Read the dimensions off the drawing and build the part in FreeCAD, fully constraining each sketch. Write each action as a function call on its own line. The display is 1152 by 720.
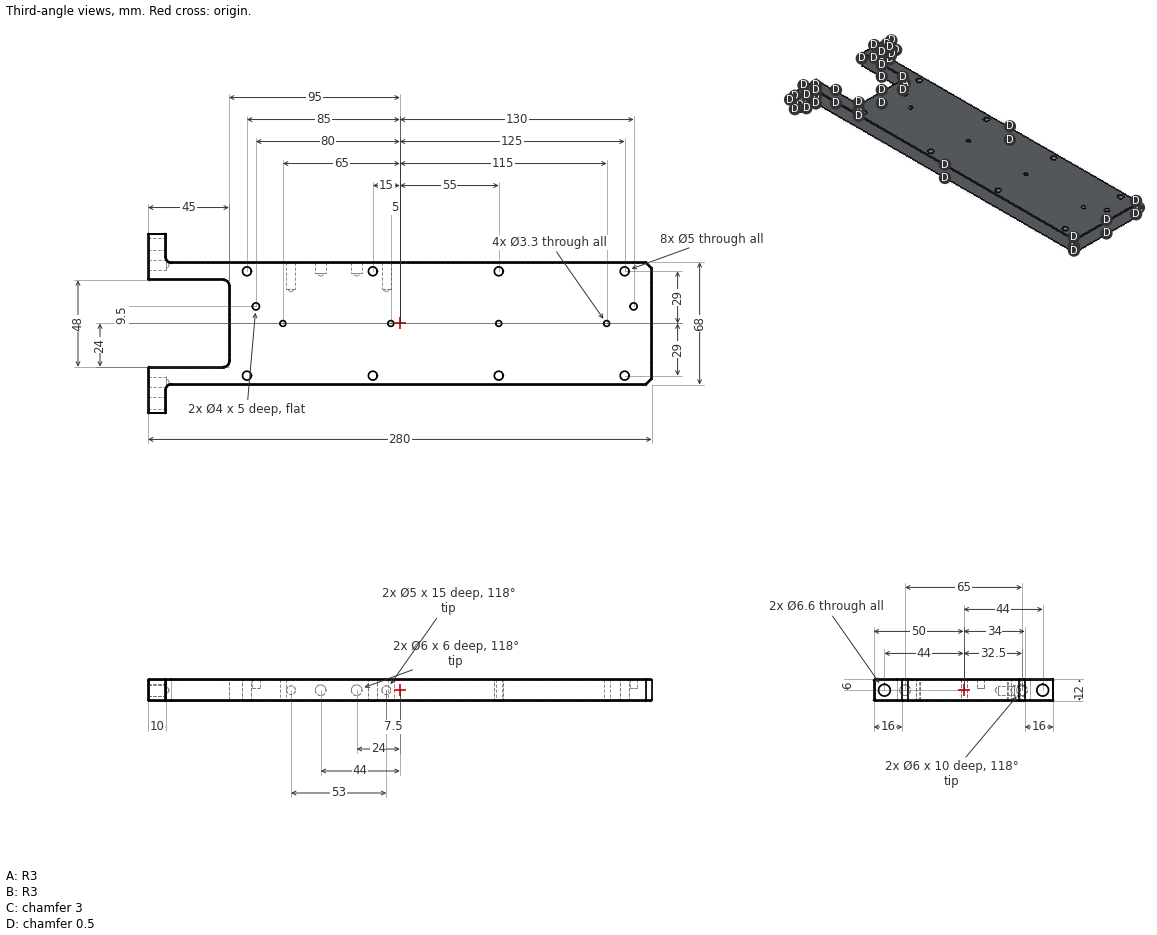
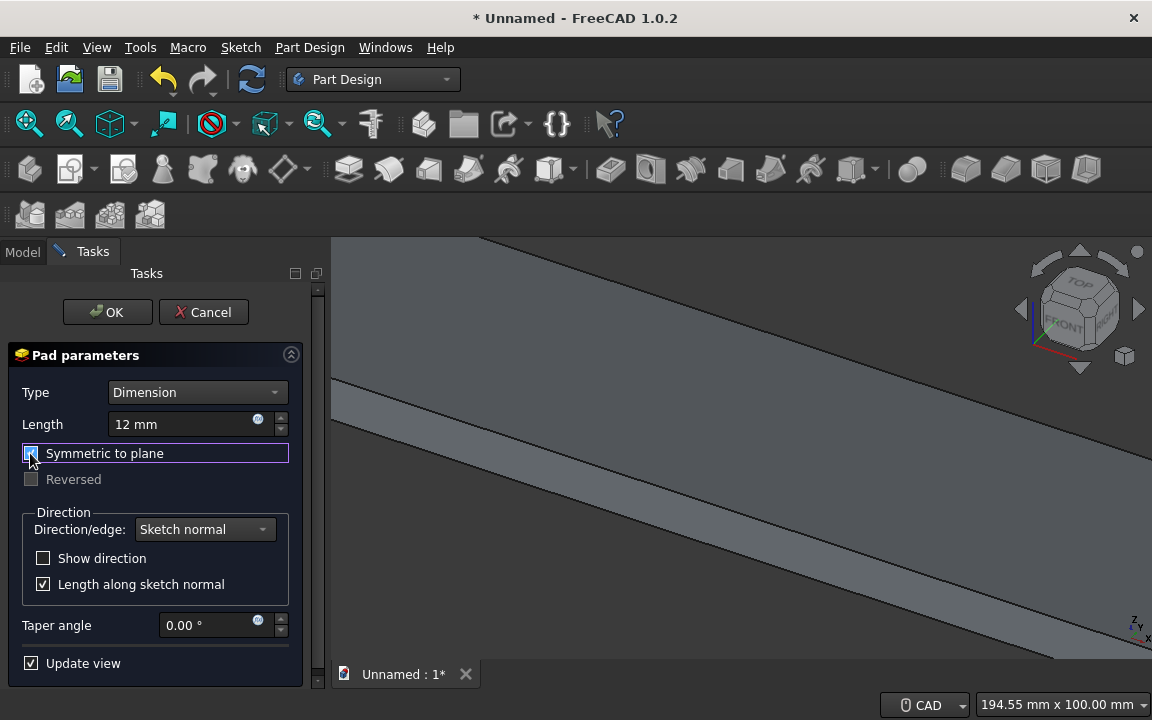
click(108, 312)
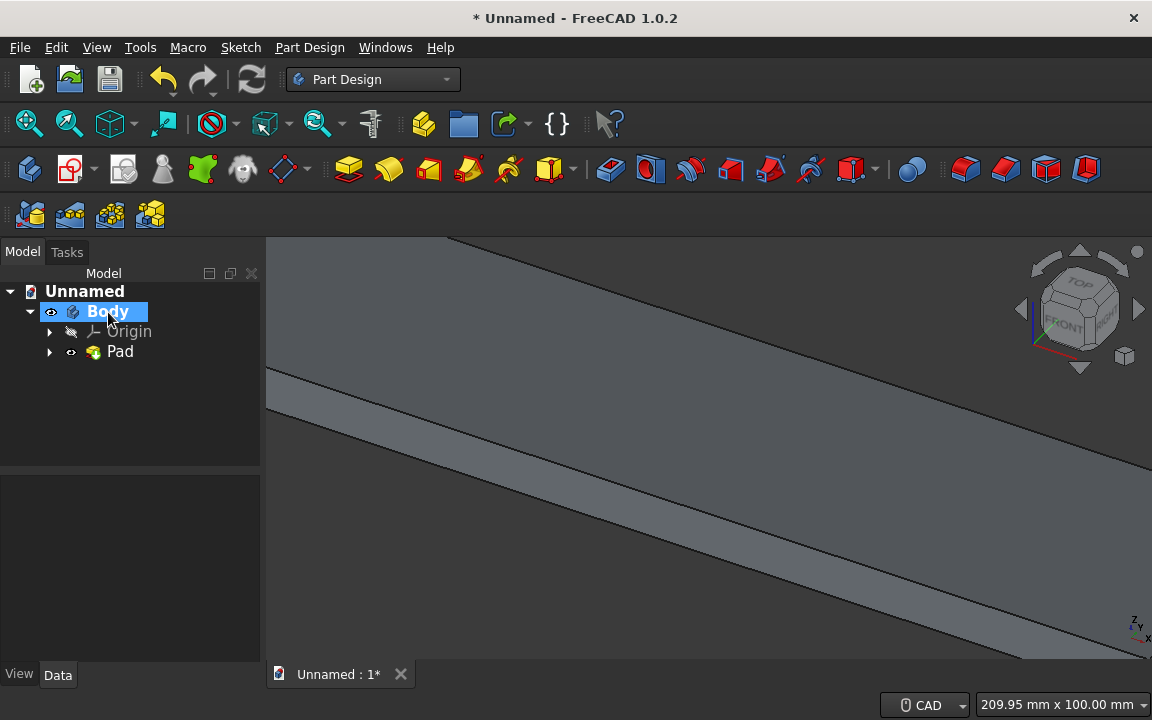
key(v)
key(f)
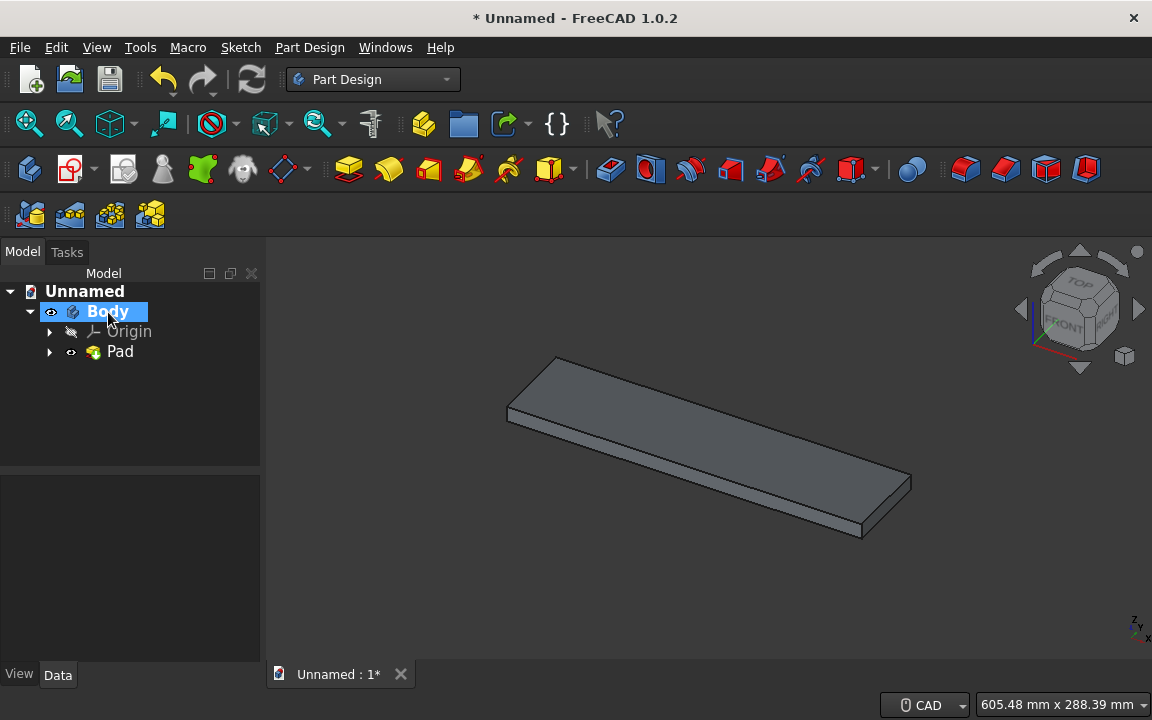
key(5)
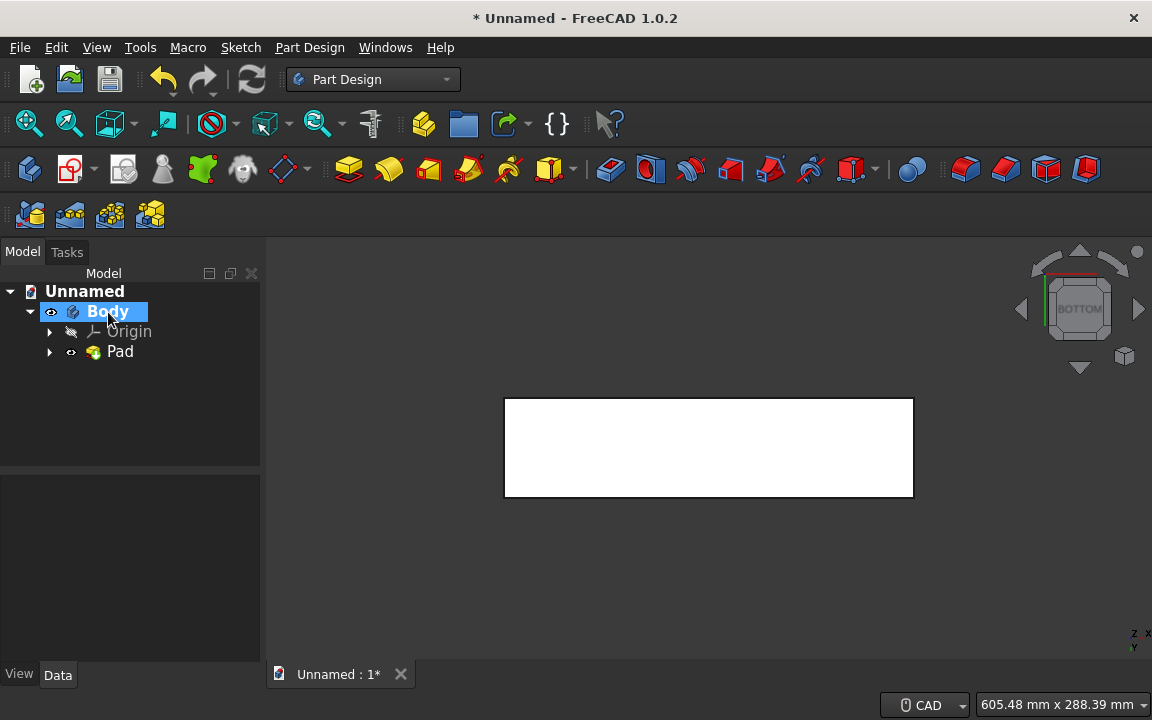
click(826, 447)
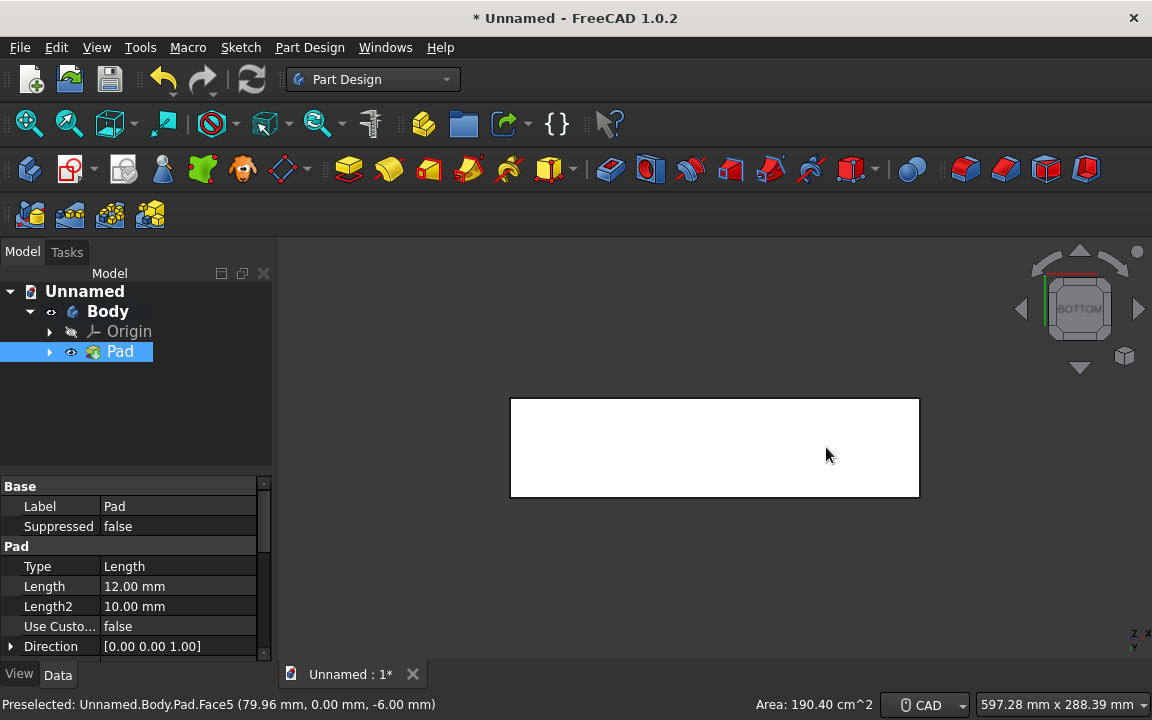
click(70, 170)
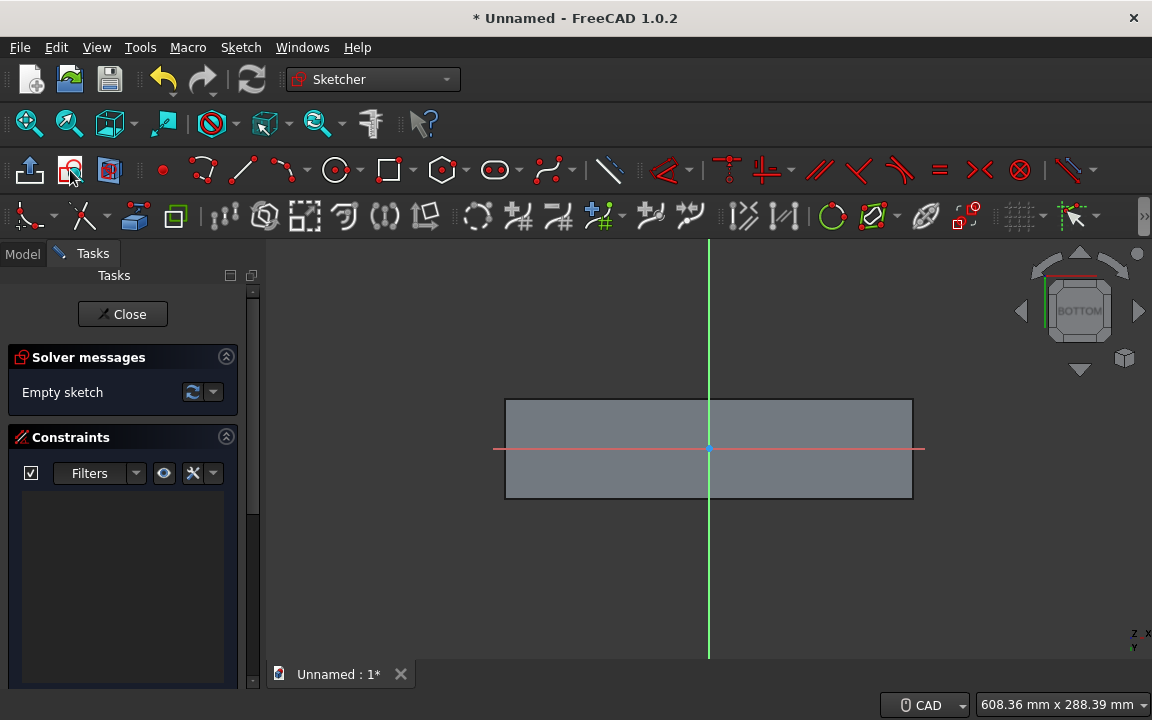
scroll(504, 449, up, 7)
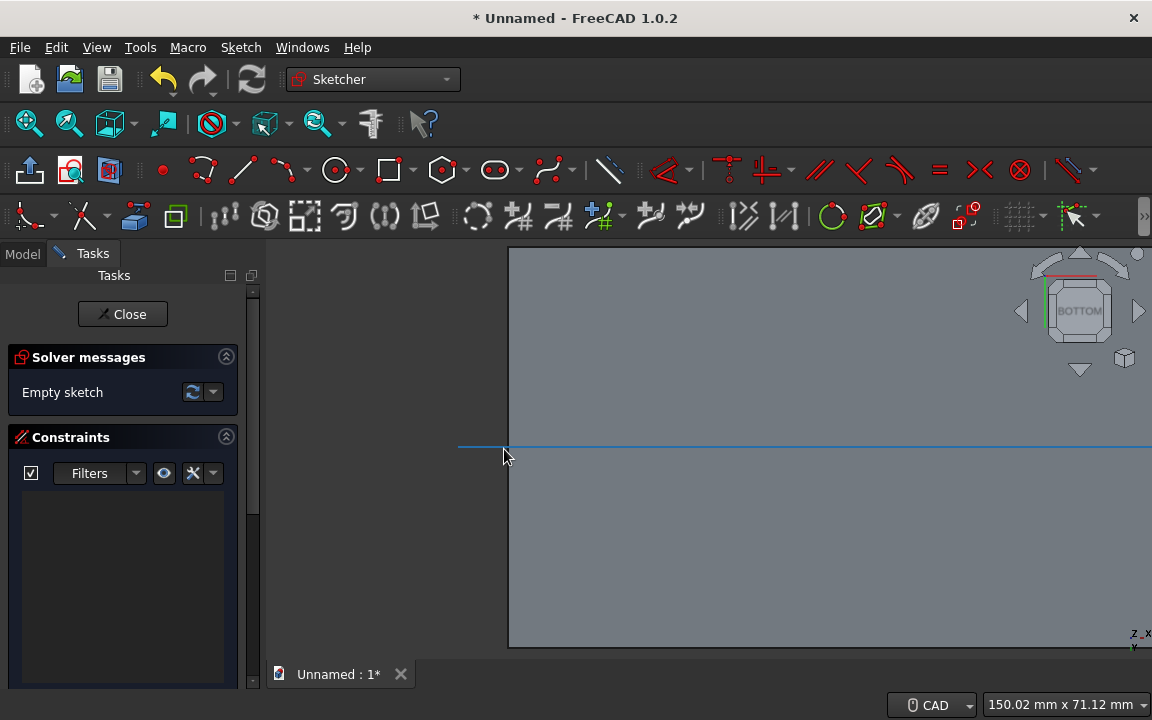
key(g)
key(r)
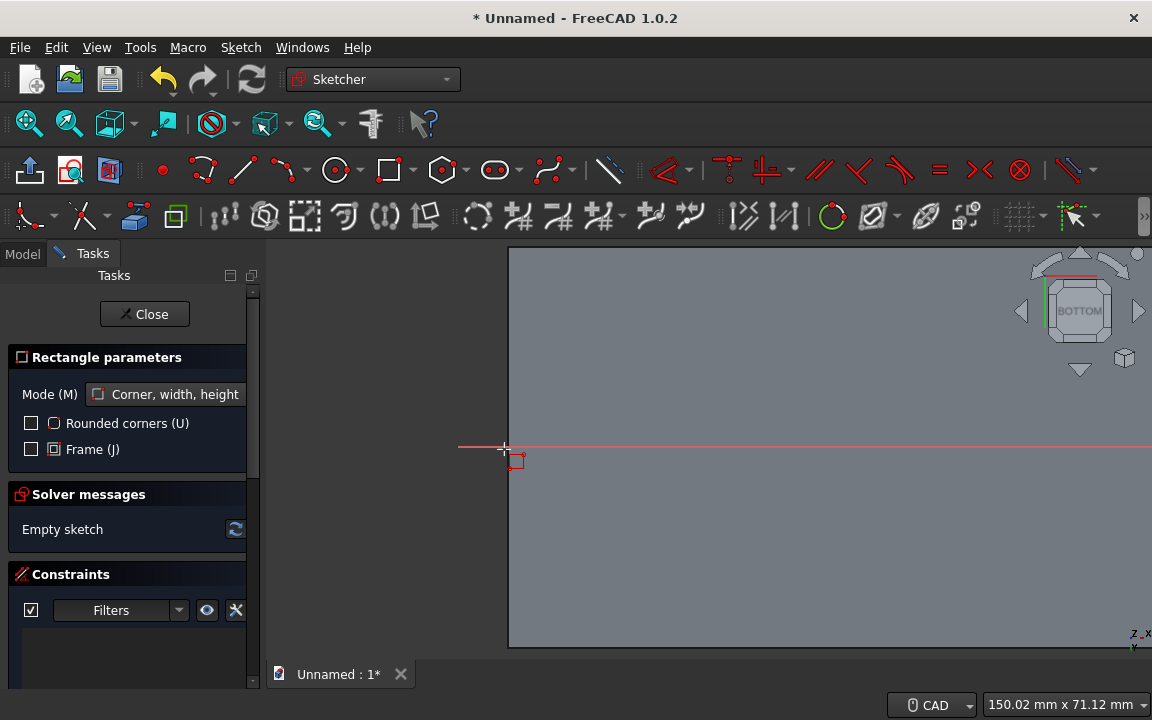
click(508, 306)
move(773, 589)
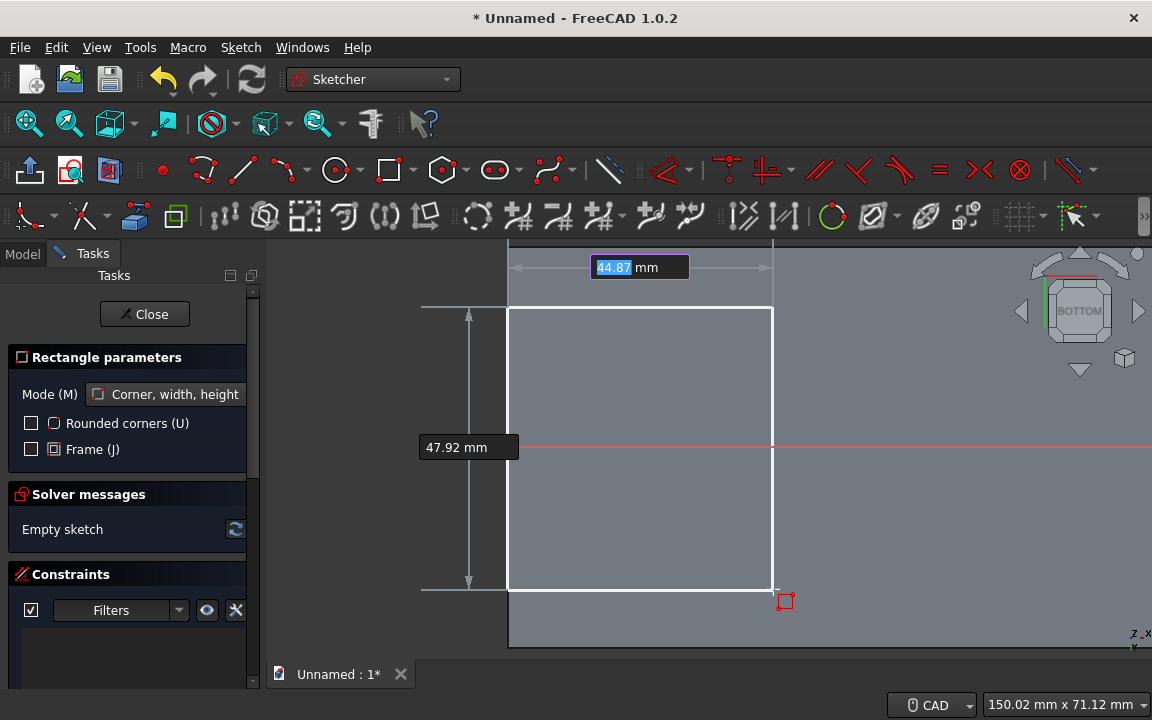
text(45)
key(Tab)
text(48)
key(Return)
key(Escape)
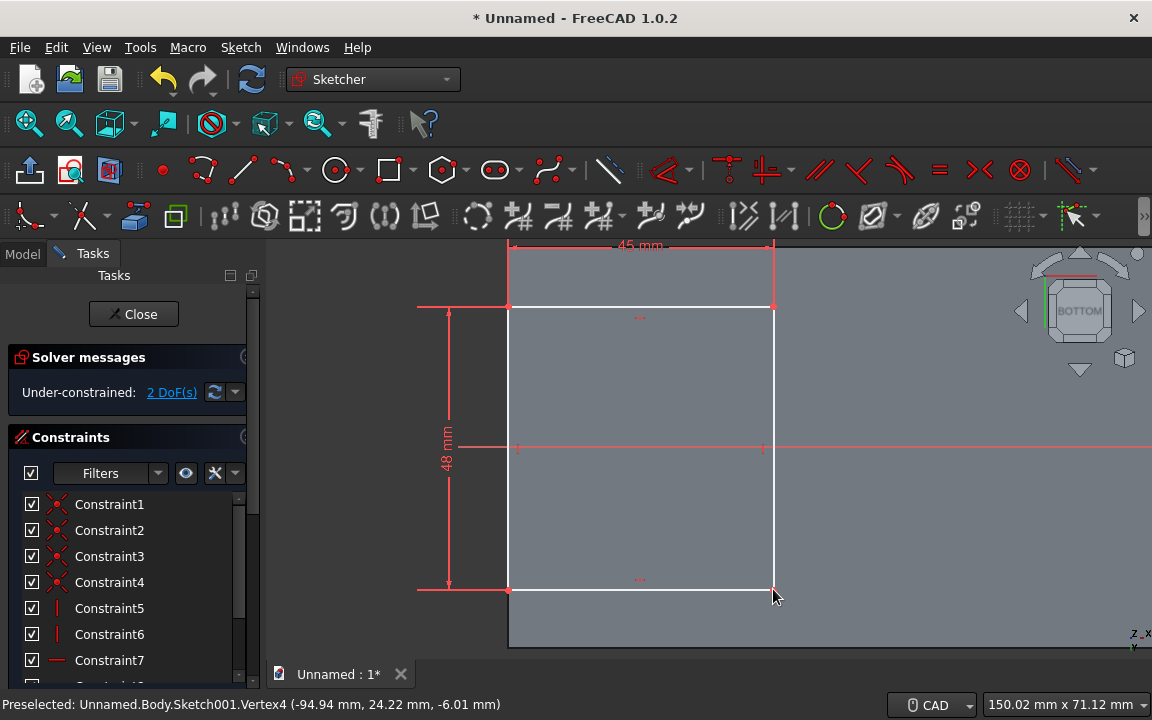
key(d)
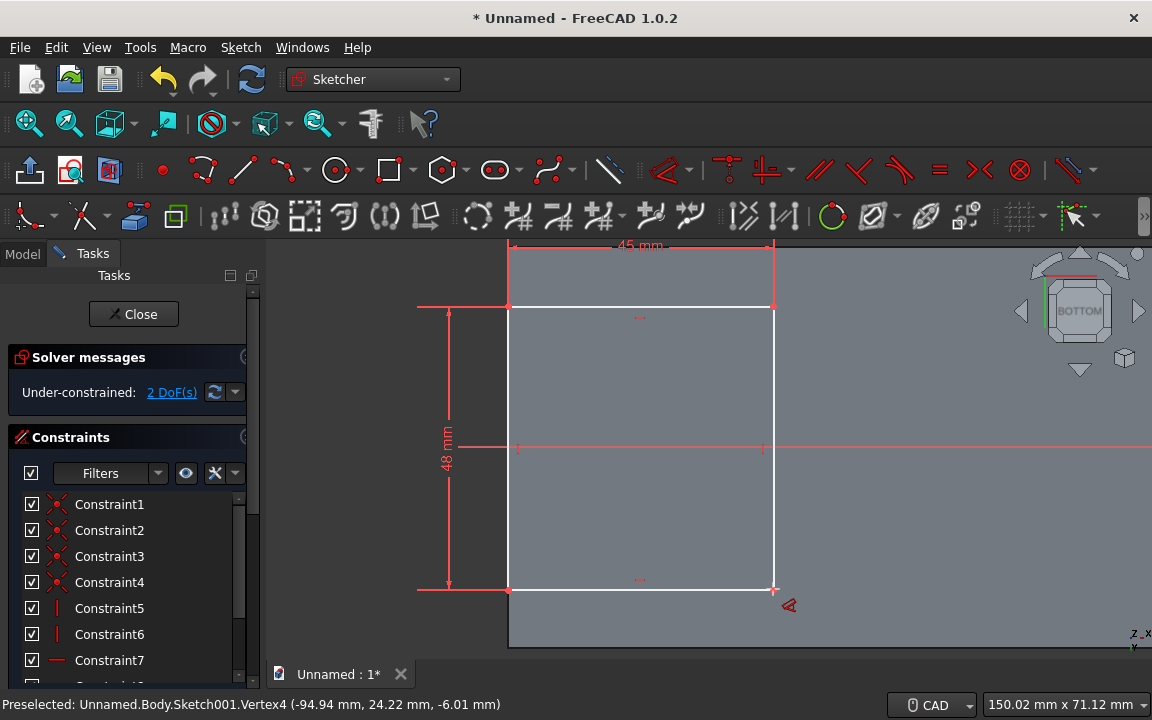
click(508, 307)
click(474, 377)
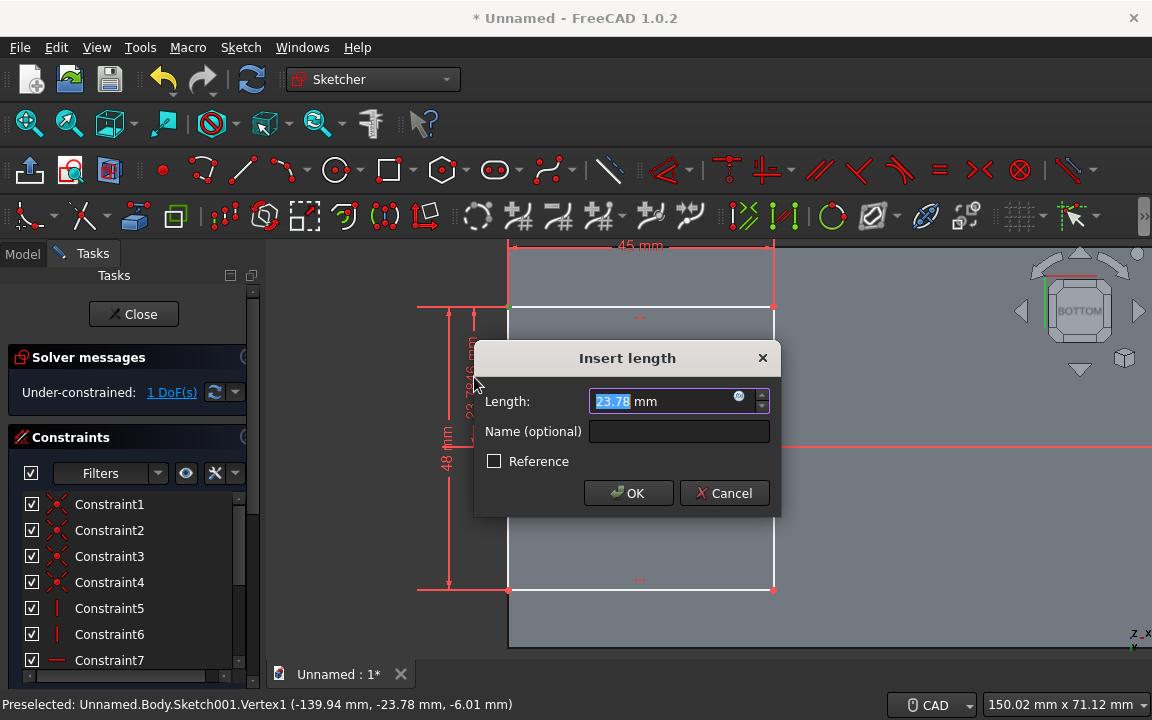
text(24)
key(Return)